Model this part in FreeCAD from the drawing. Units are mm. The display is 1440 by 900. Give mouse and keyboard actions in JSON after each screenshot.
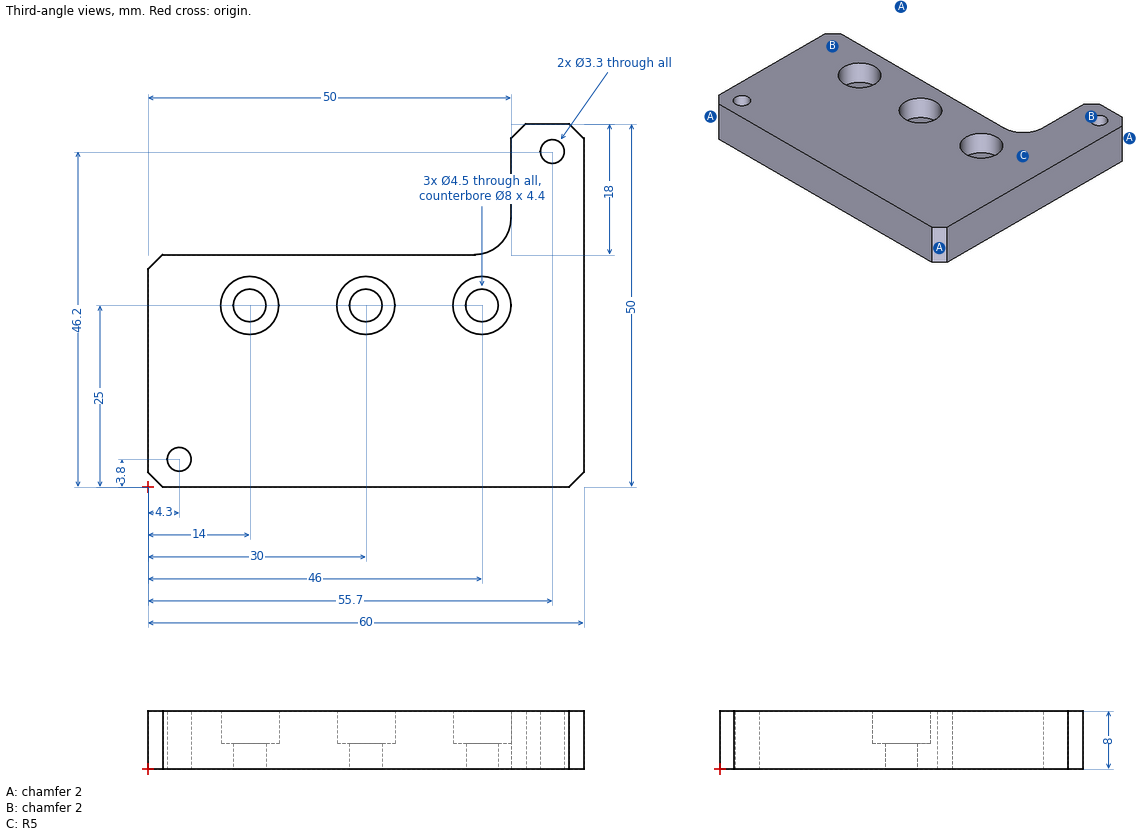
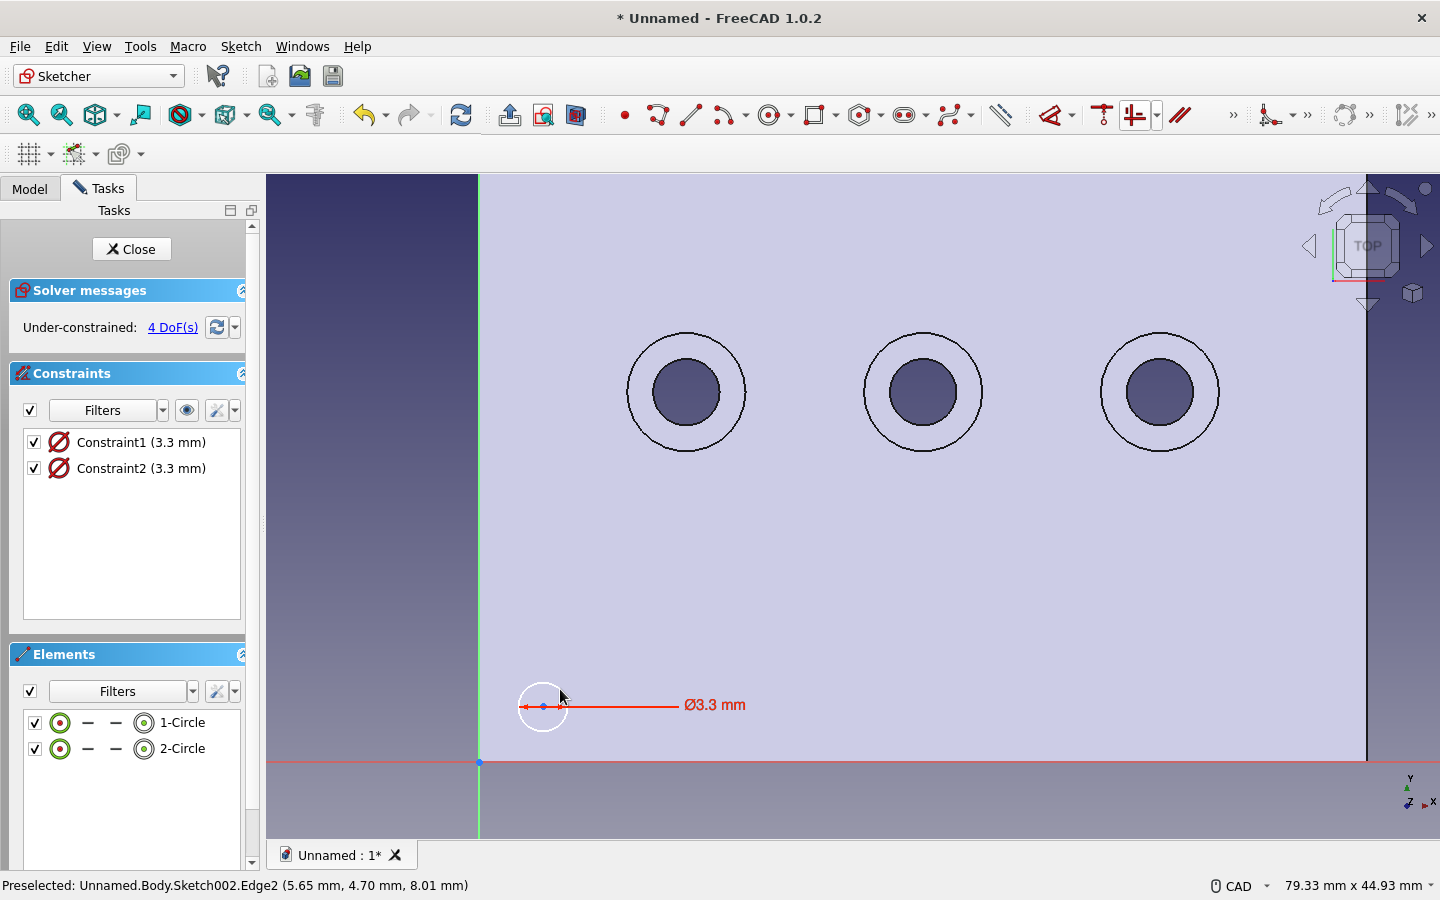
{"action": "left_click", "coordinate": [1050, 116]}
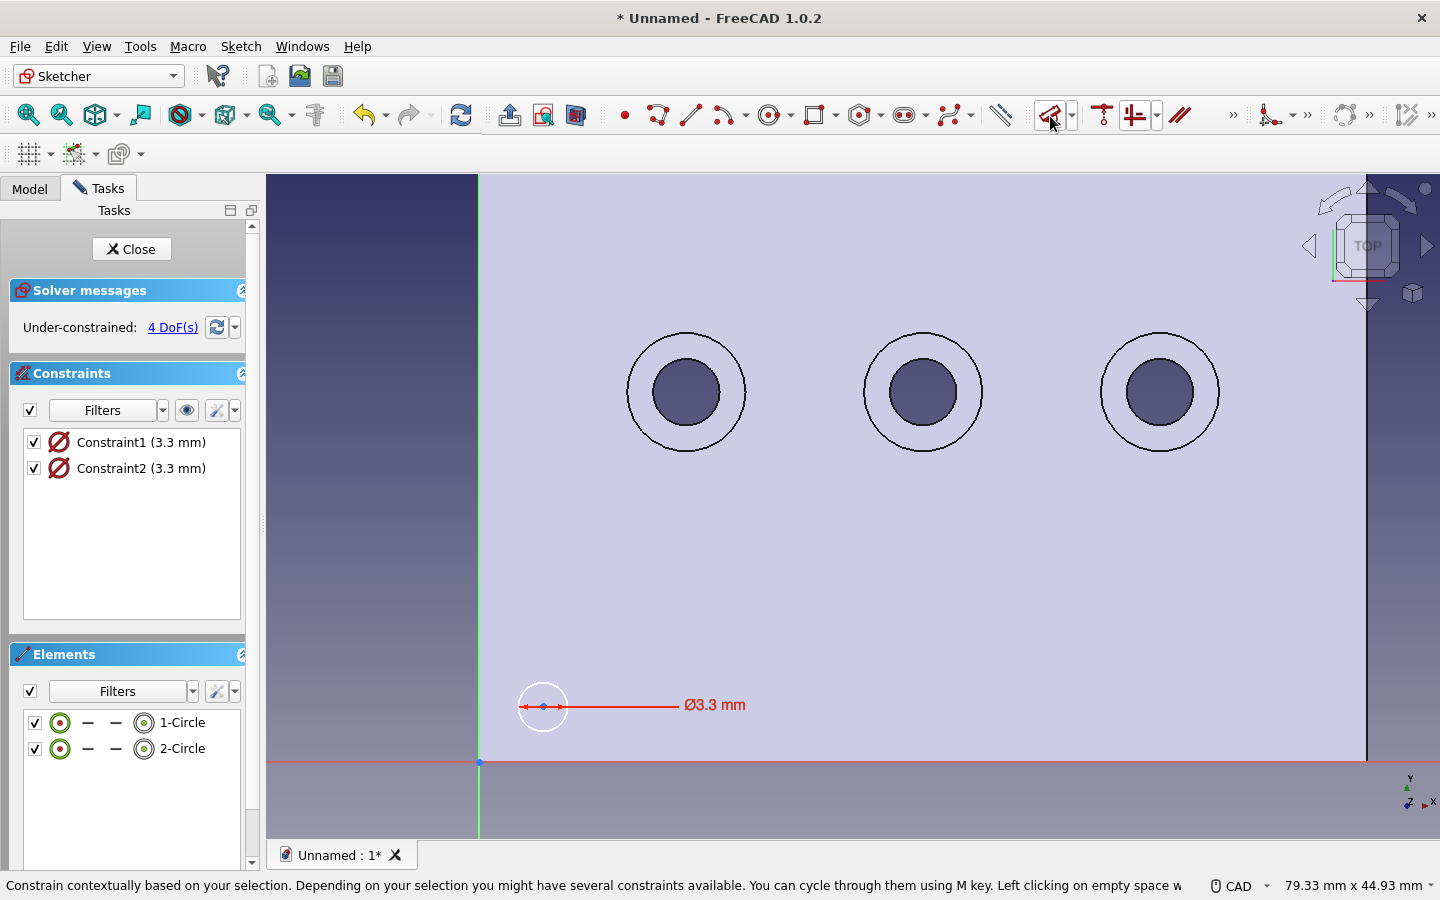
{"action": "left_click", "coordinate": [543, 707]}
{"action": "left_click", "coordinate": [511, 796]}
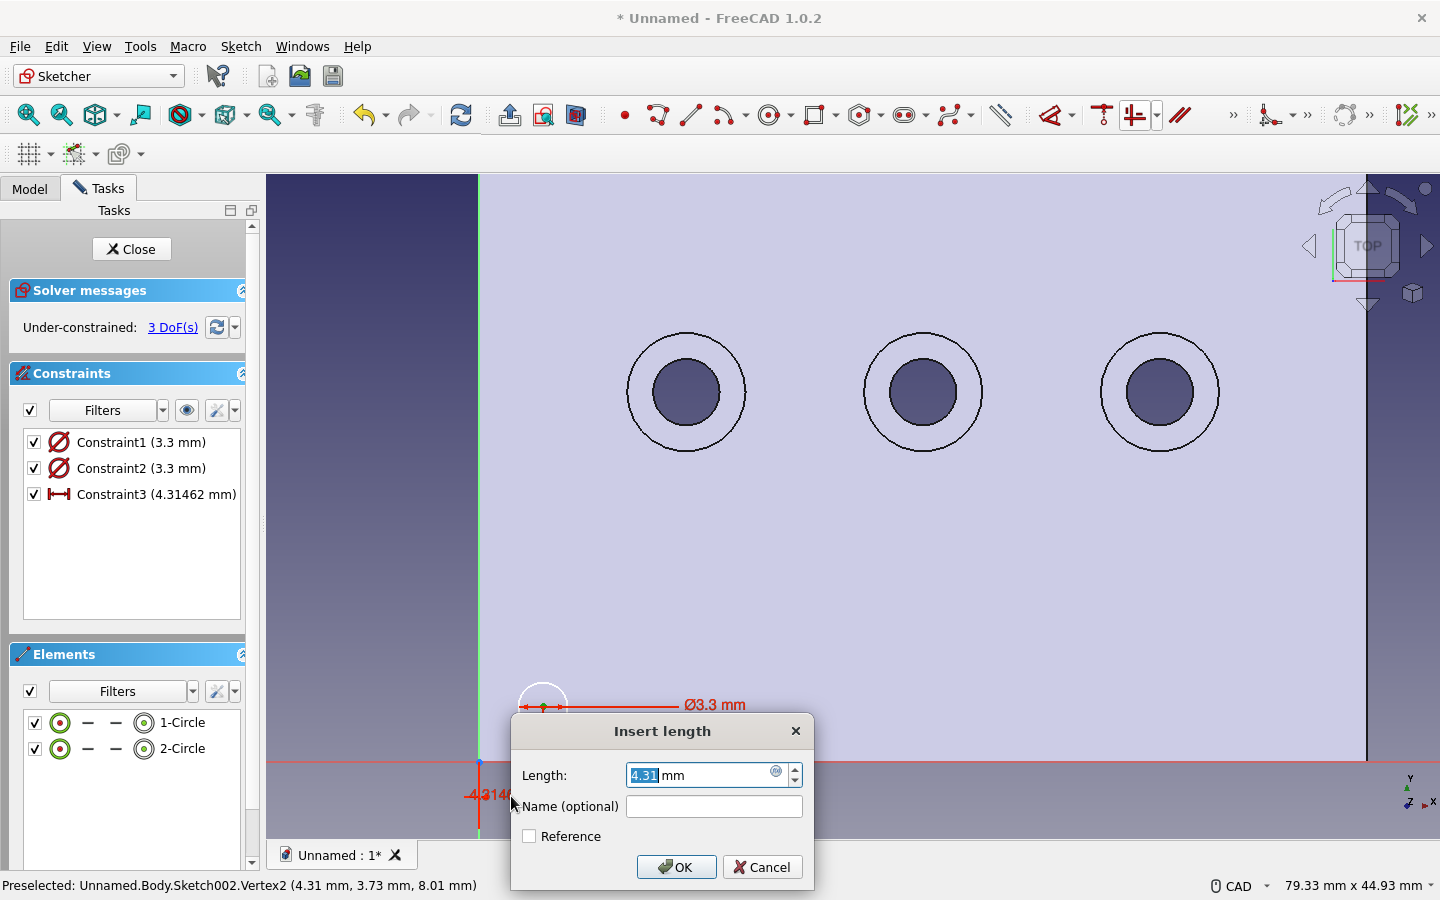
{"action": "type", "text": "4.3"}
{"action": "key", "text": "Return"}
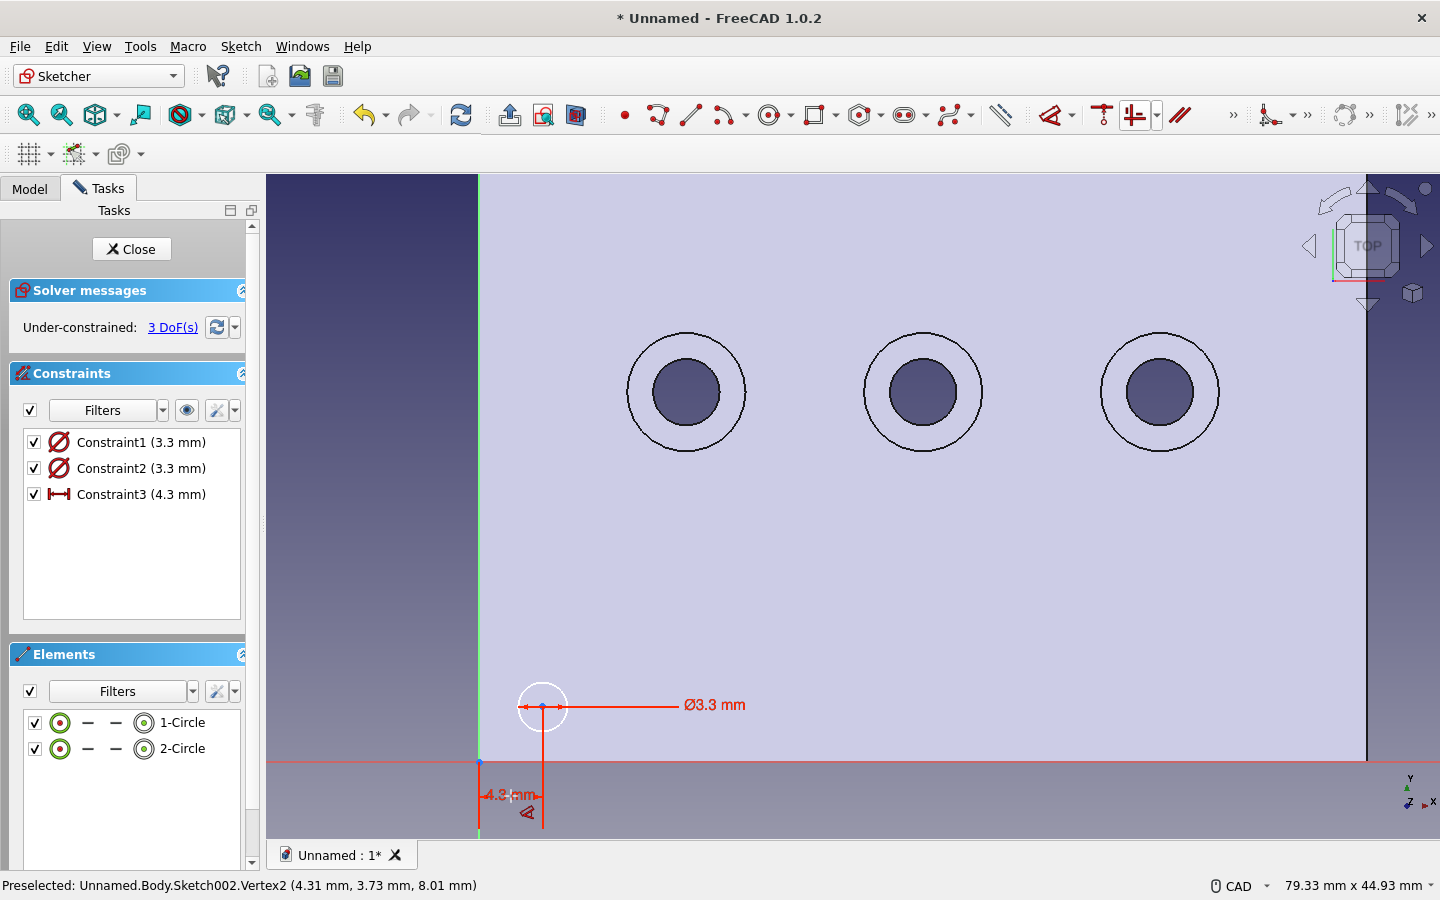
{"action": "left_click", "coordinate": [543, 707]}
{"action": "left_click", "coordinate": [445, 735]}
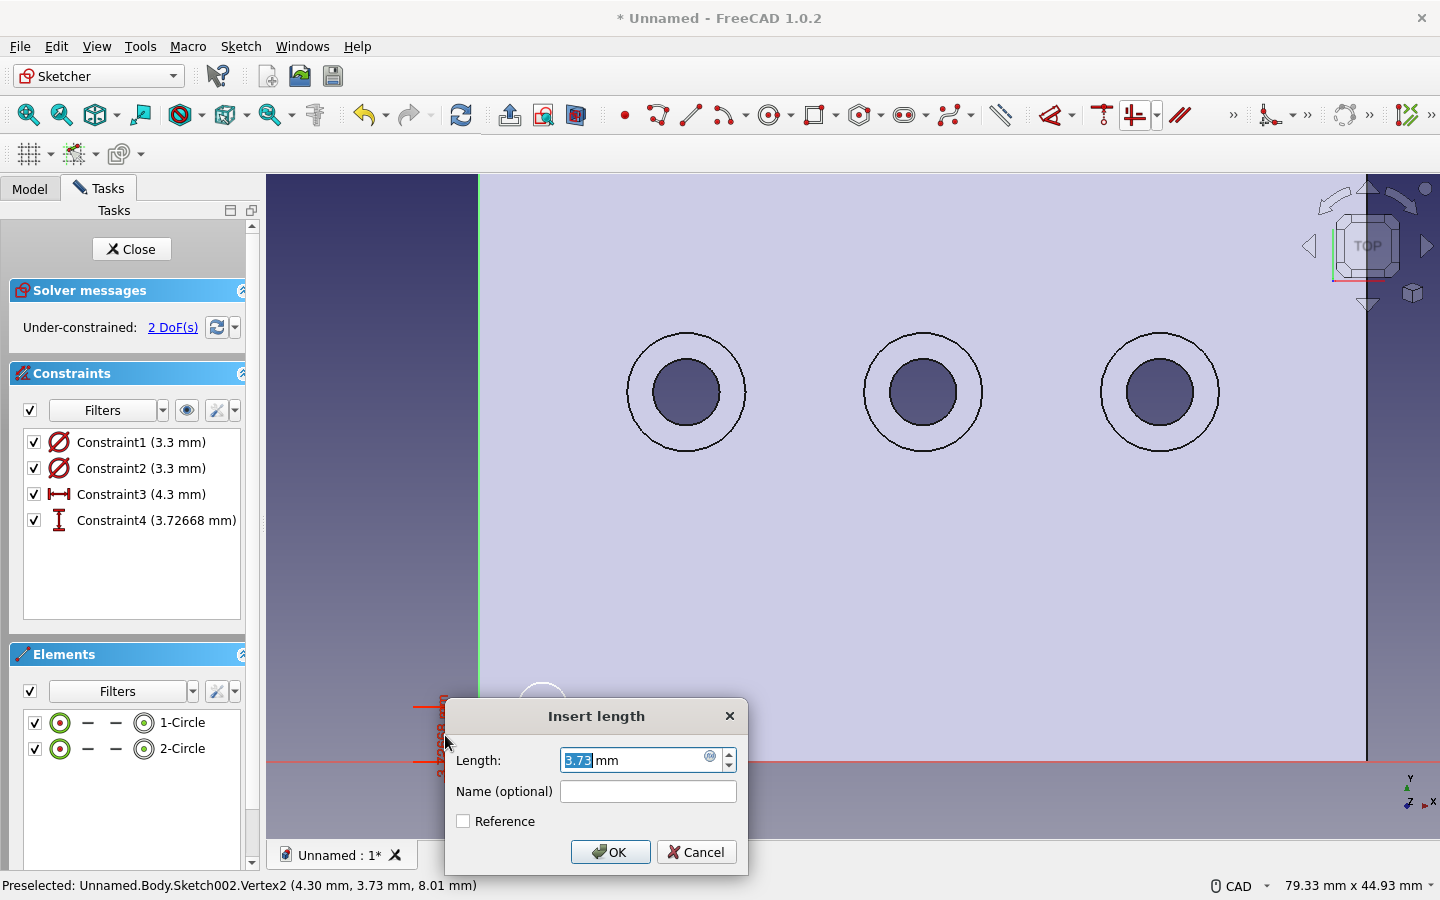
{"action": "type", "text": "3.8"}
{"action": "key", "text": "Return"}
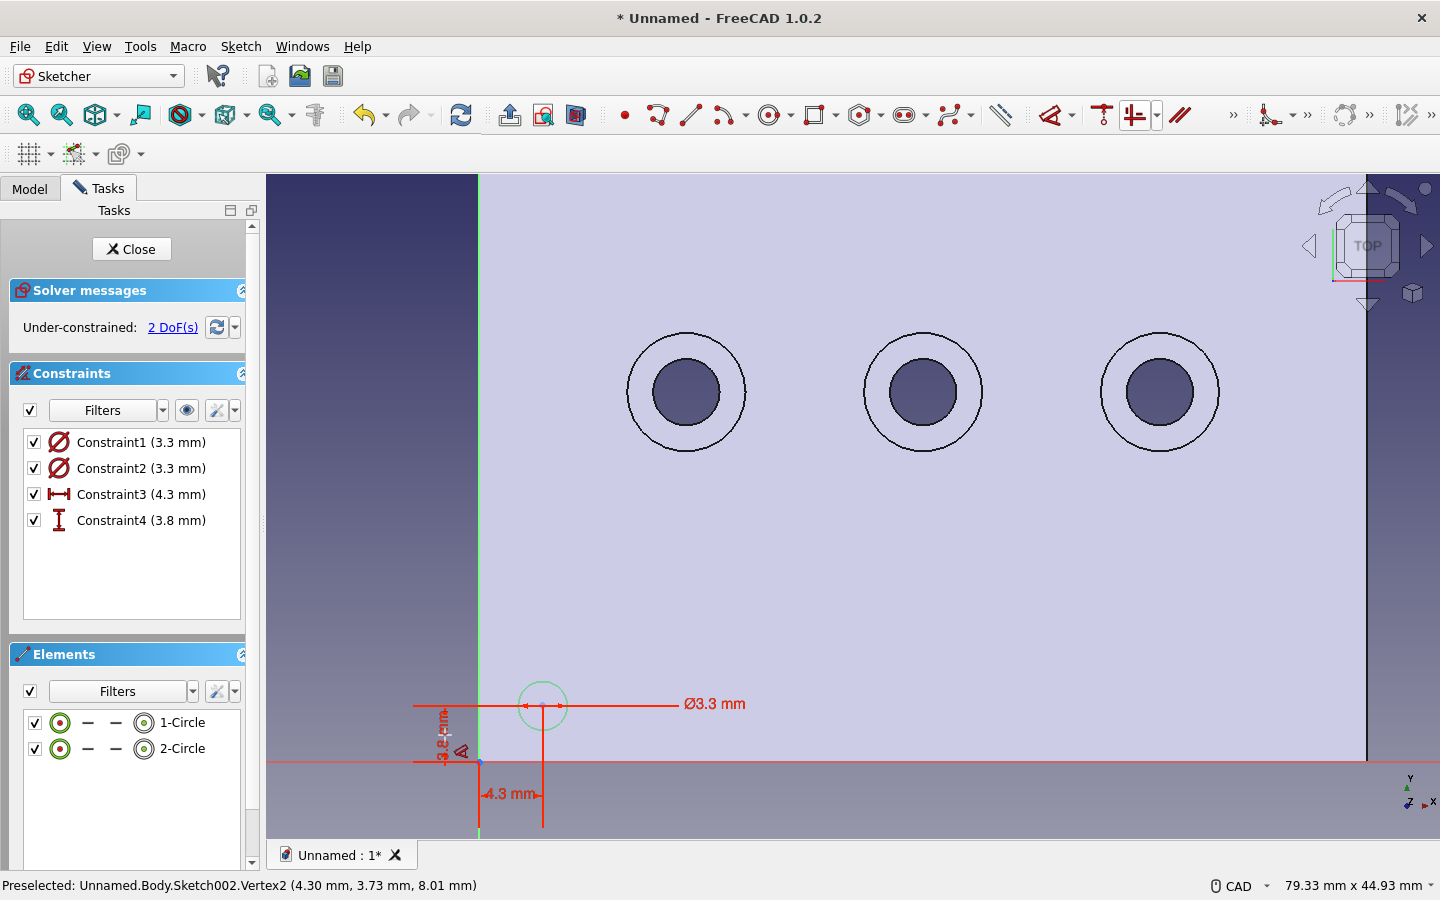
{"action": "scroll", "coordinate": [542, 707], "scroll_direction": "down", "scroll_amount": 2}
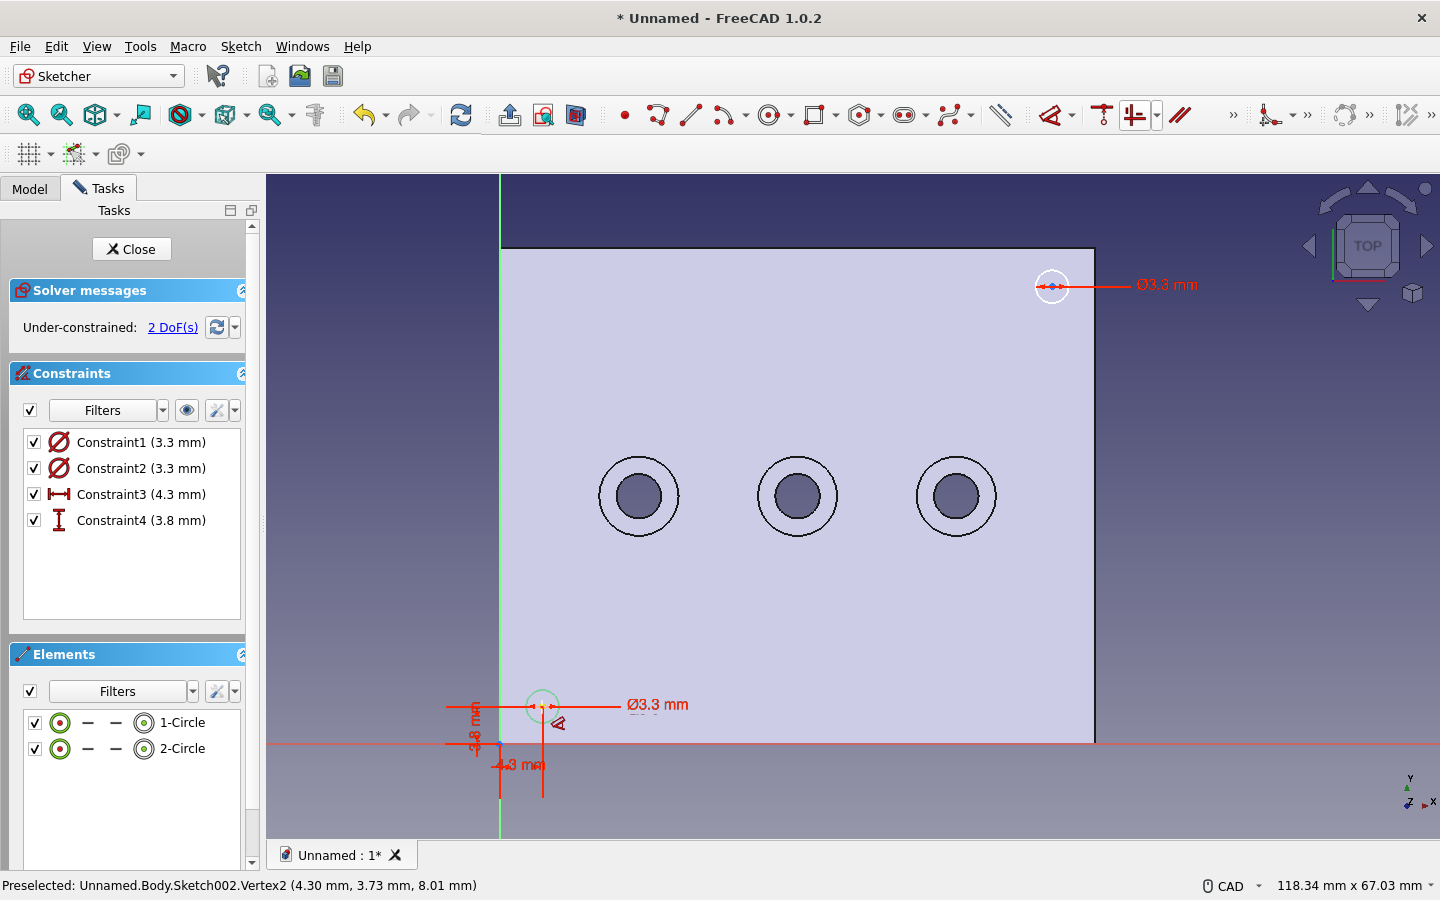
{"action": "left_click", "coordinate": [1052, 287]}
{"action": "left_click", "coordinate": [776, 778]}